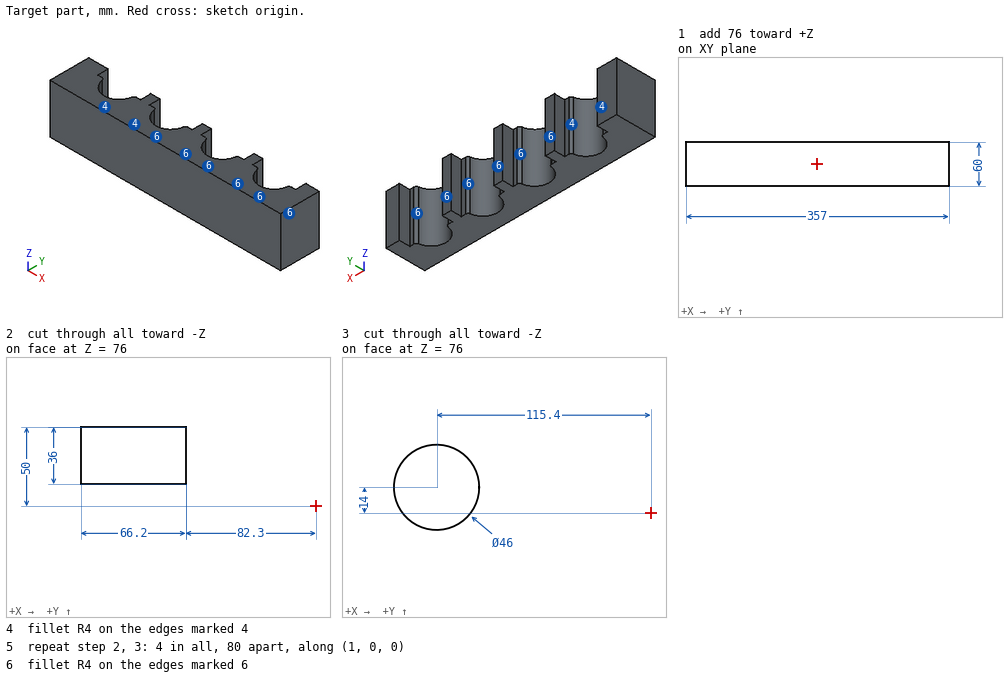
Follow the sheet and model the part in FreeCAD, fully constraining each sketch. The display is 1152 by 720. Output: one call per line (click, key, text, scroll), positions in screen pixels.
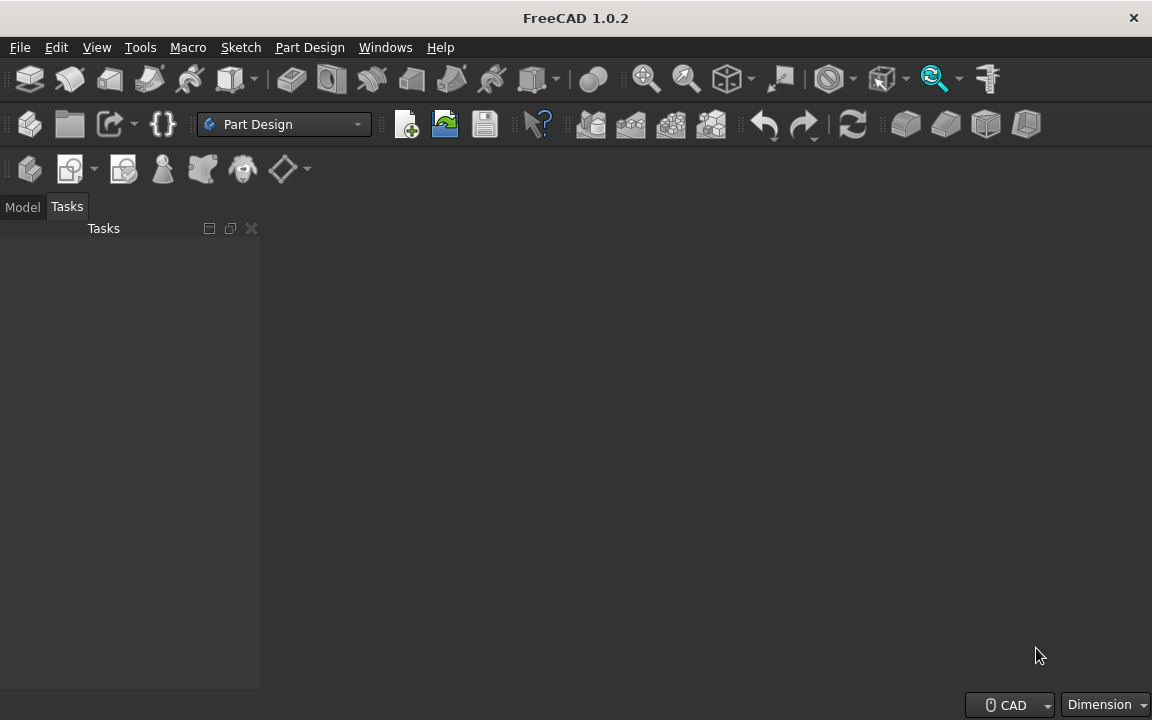
click(406, 124)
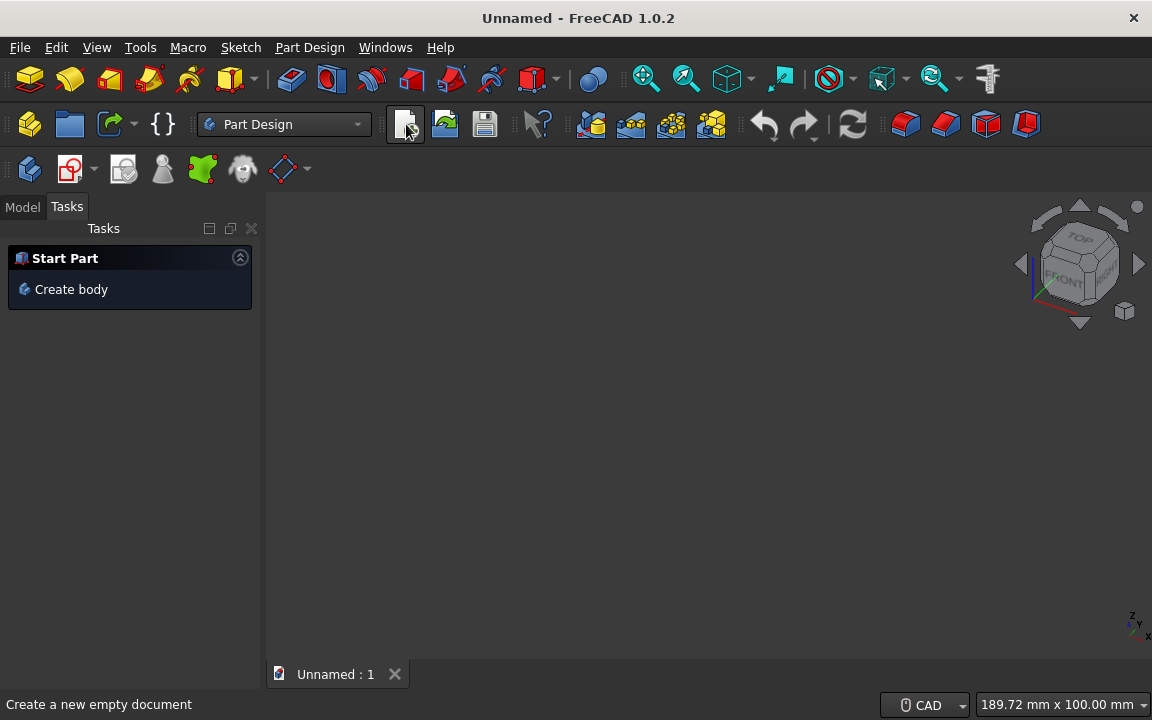
click(70, 170)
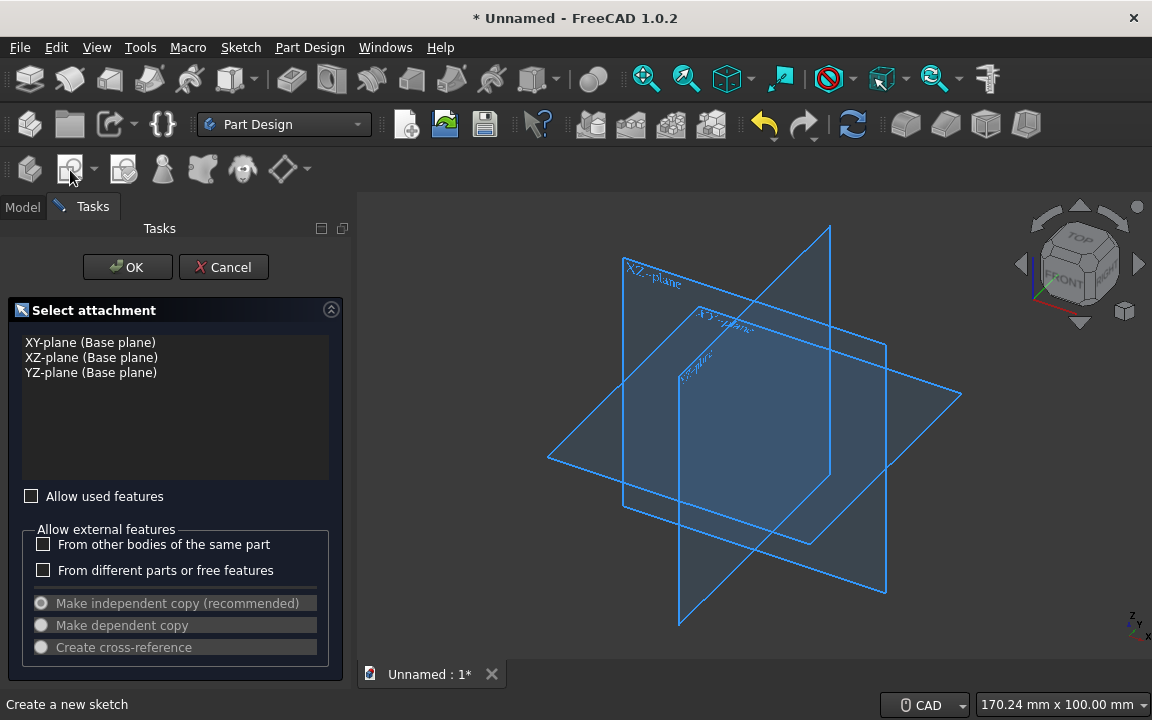
click(82, 342)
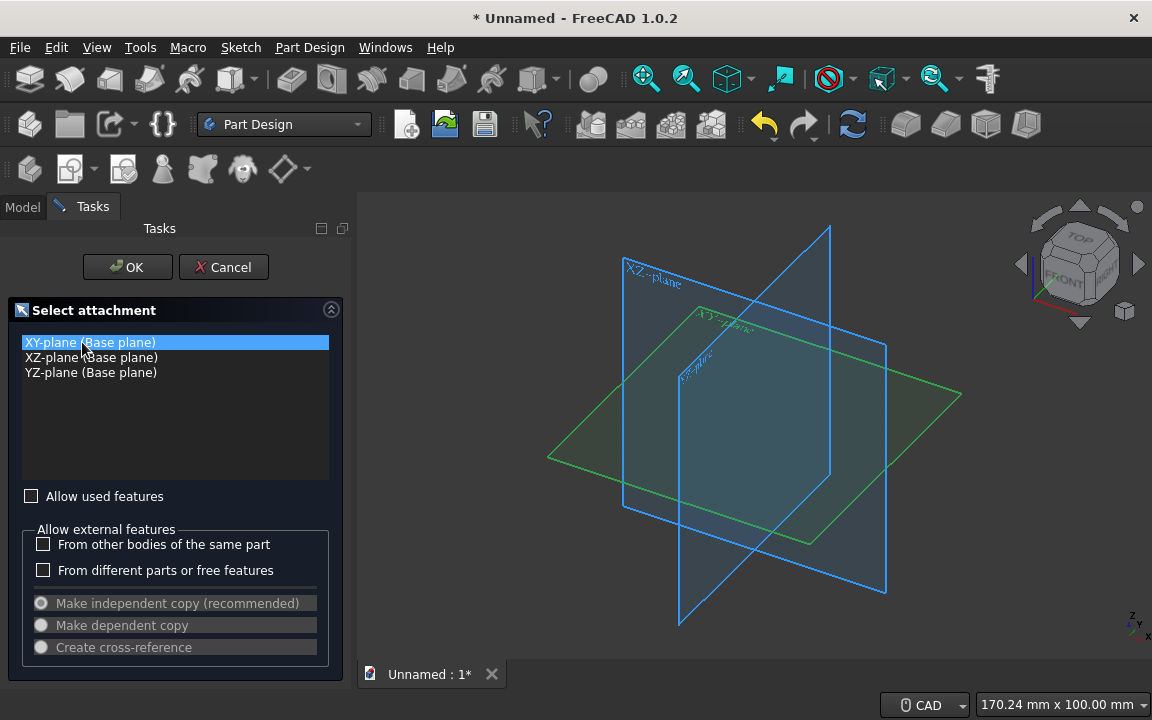
click(128, 267)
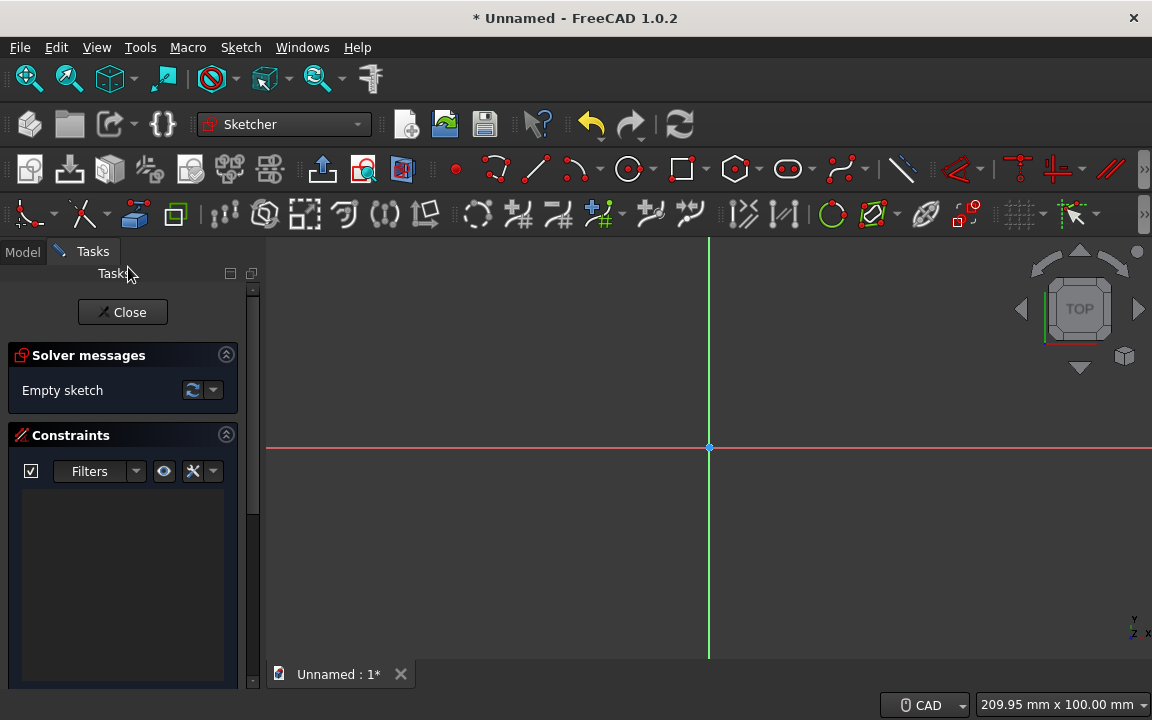
scroll(611, 448, down, 6)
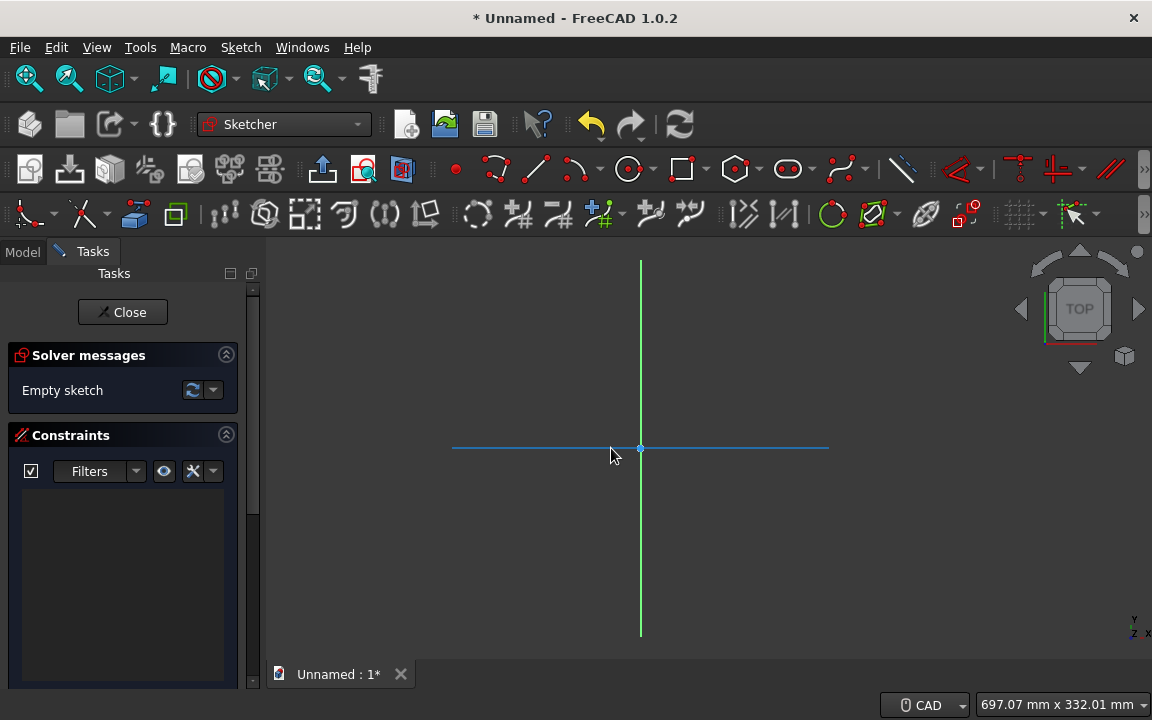
key(g)
key(v)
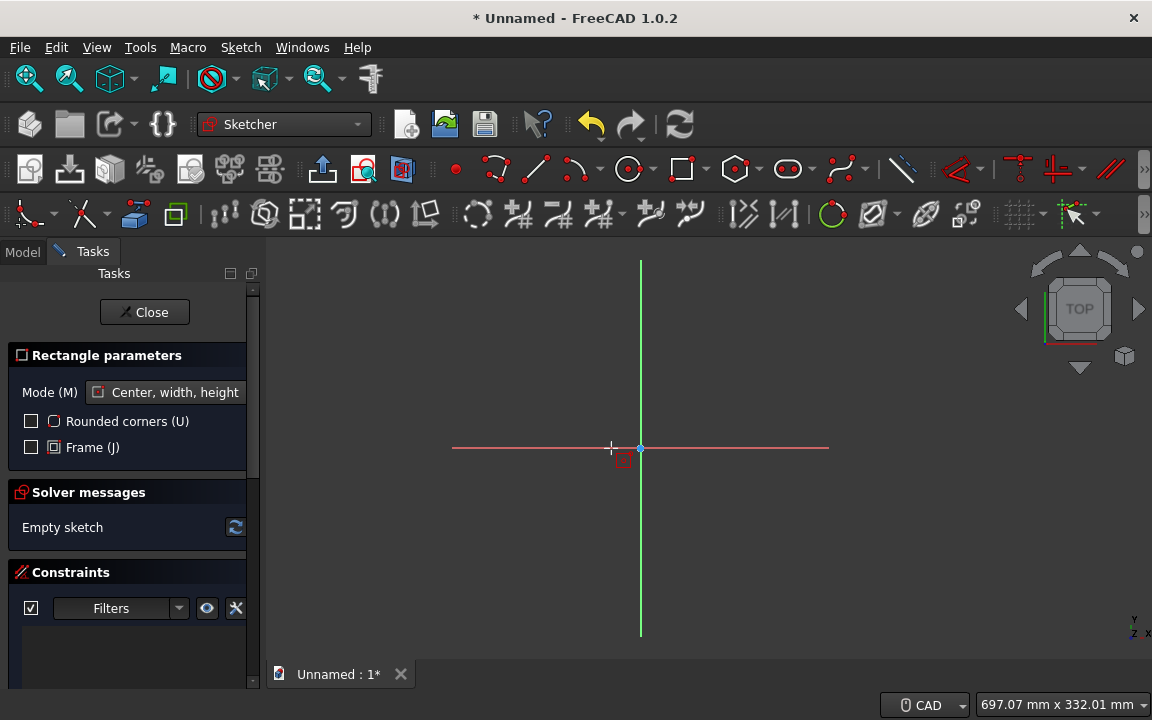
click(641, 448)
move(868, 410)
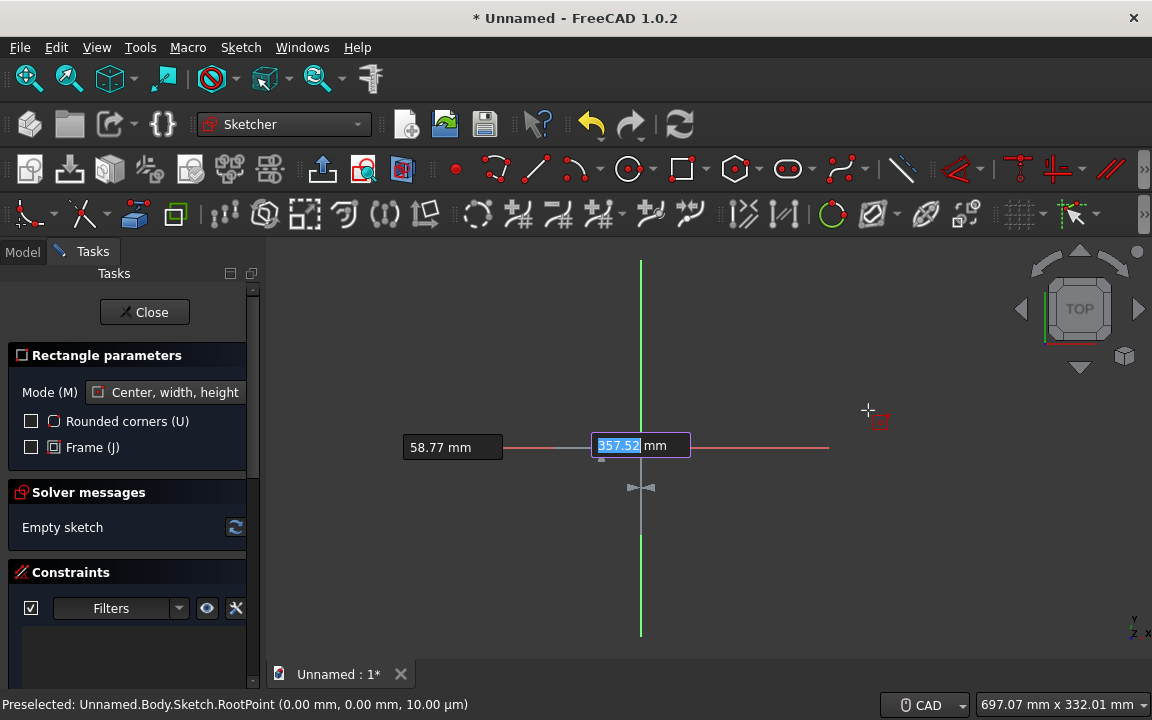
text(357)
key(Tab)
text(60)
key(Return)
key(Escape)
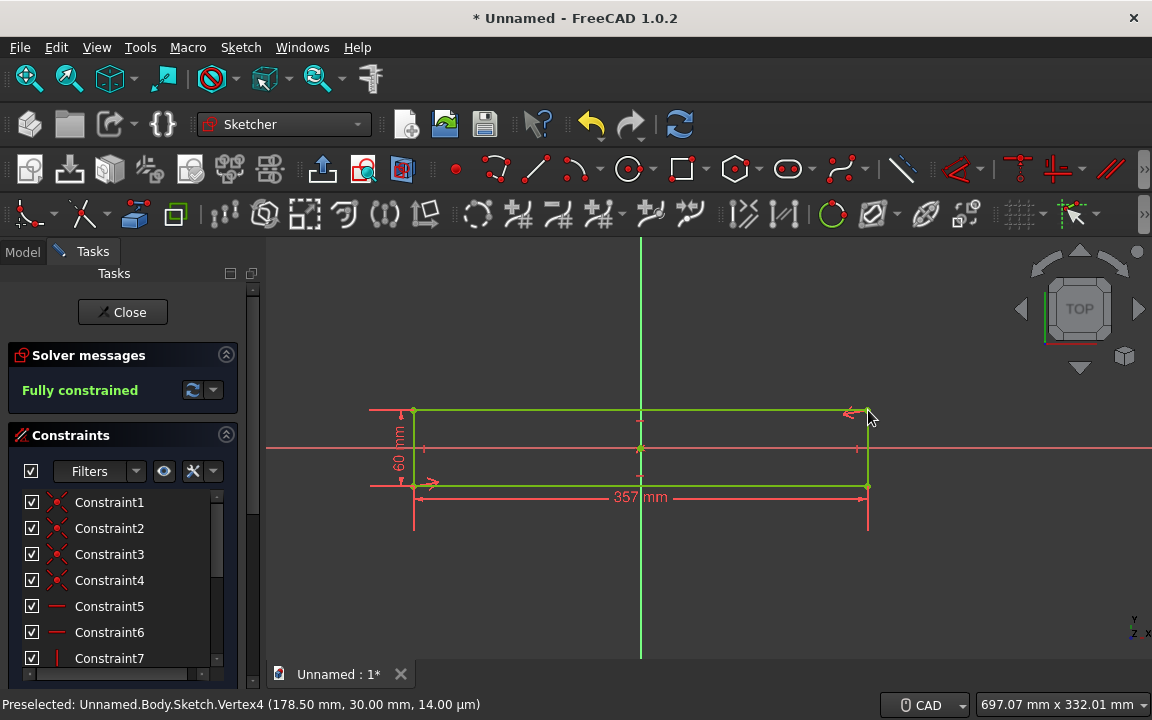
click(123, 312)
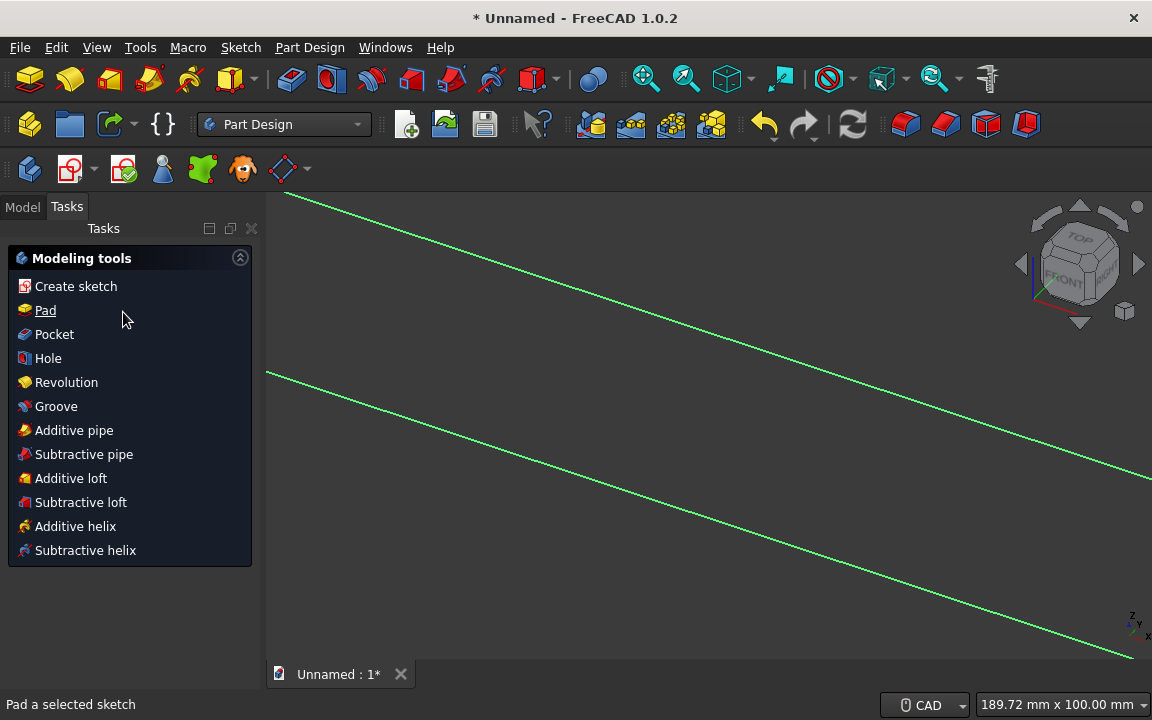
click(30, 80)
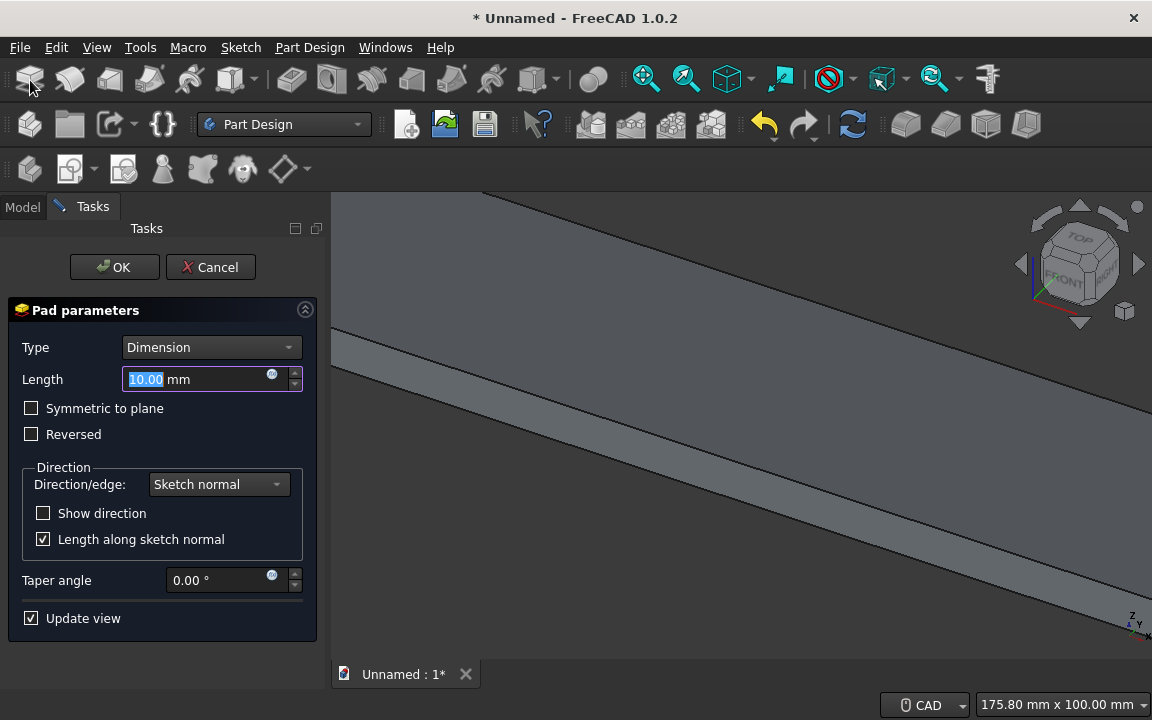
text(76)
key(Tab)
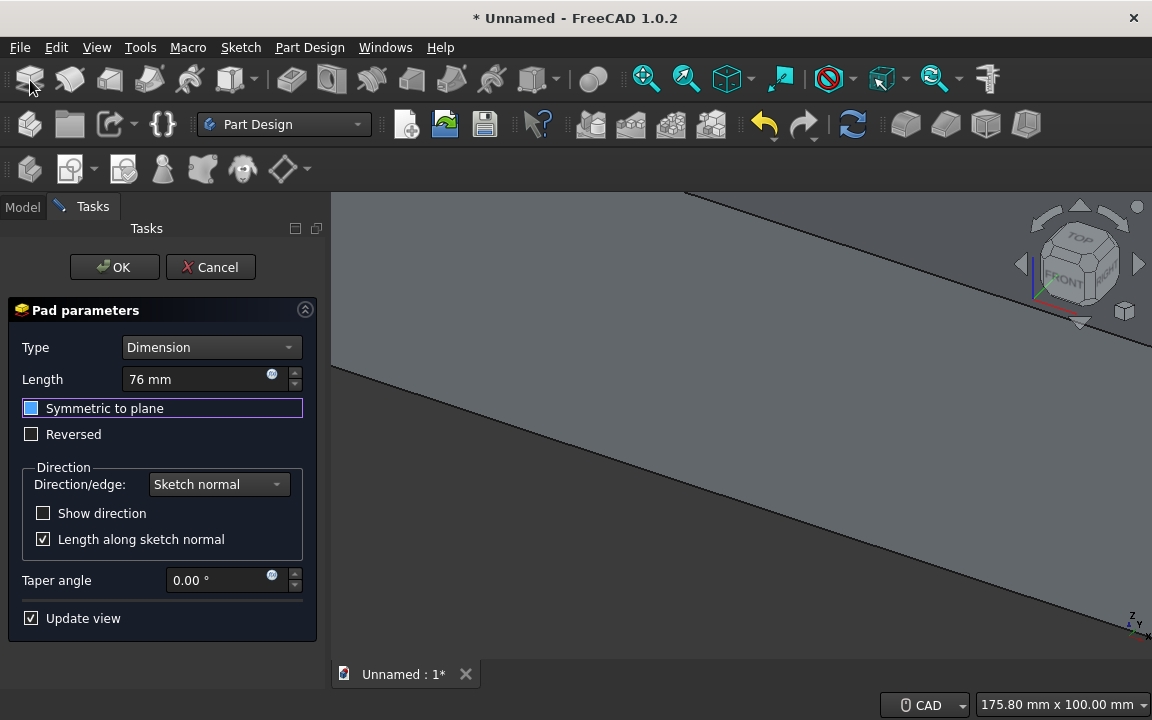
click(115, 267)